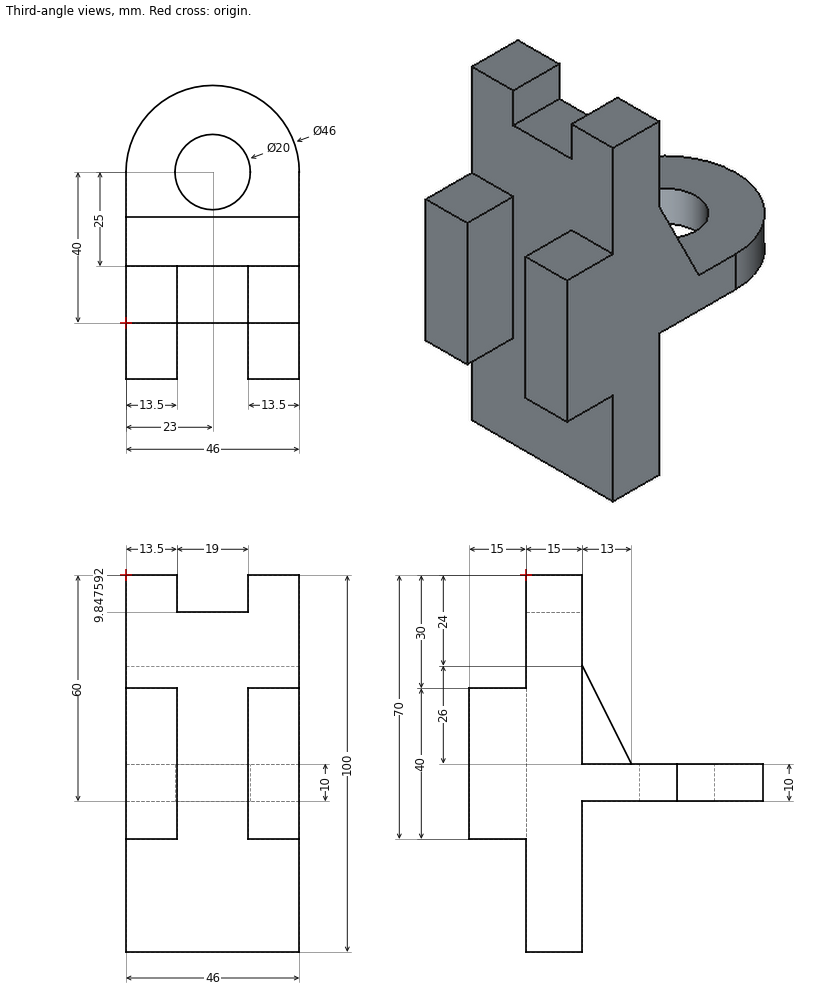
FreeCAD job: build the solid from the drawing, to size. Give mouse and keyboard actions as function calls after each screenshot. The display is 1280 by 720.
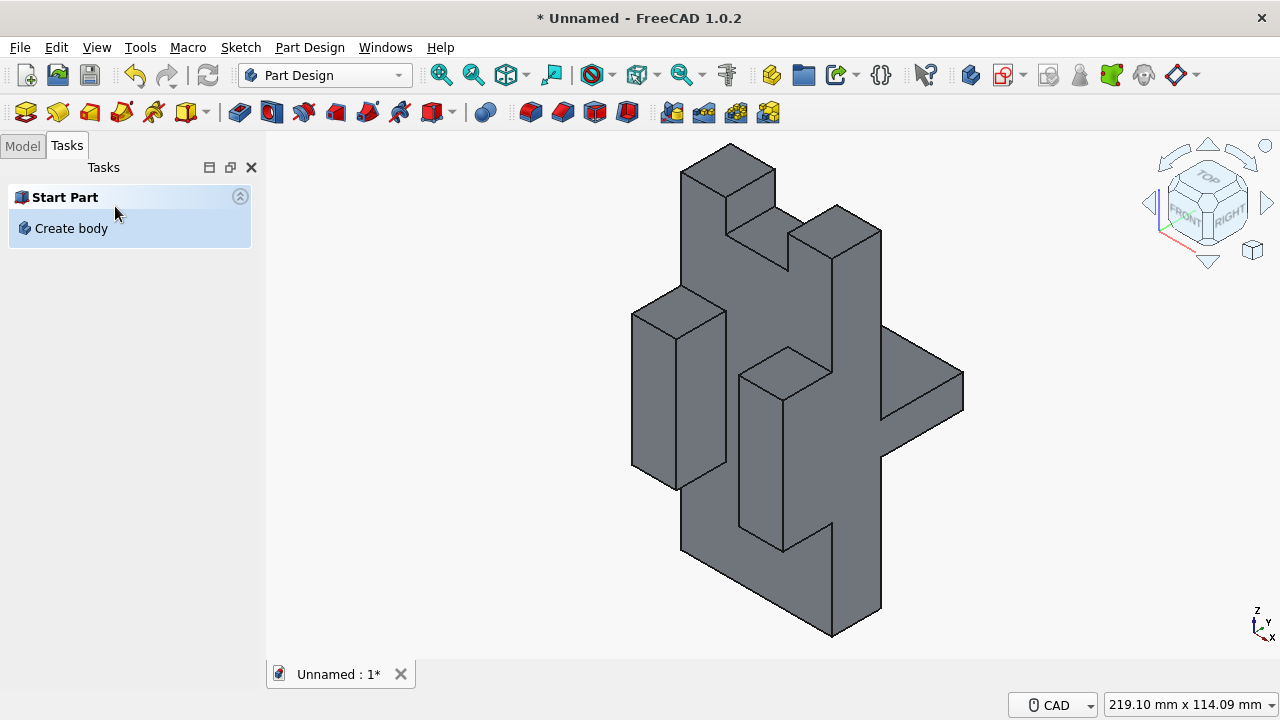
click(442, 76)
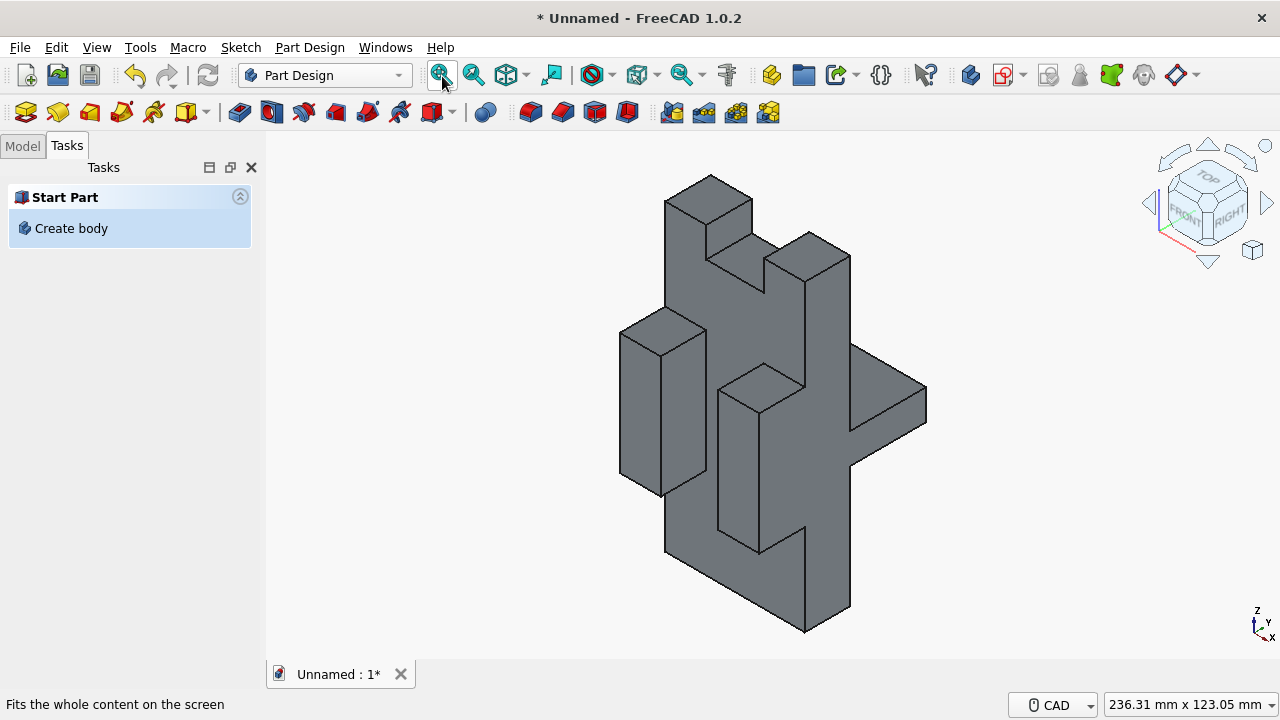
click(869, 384)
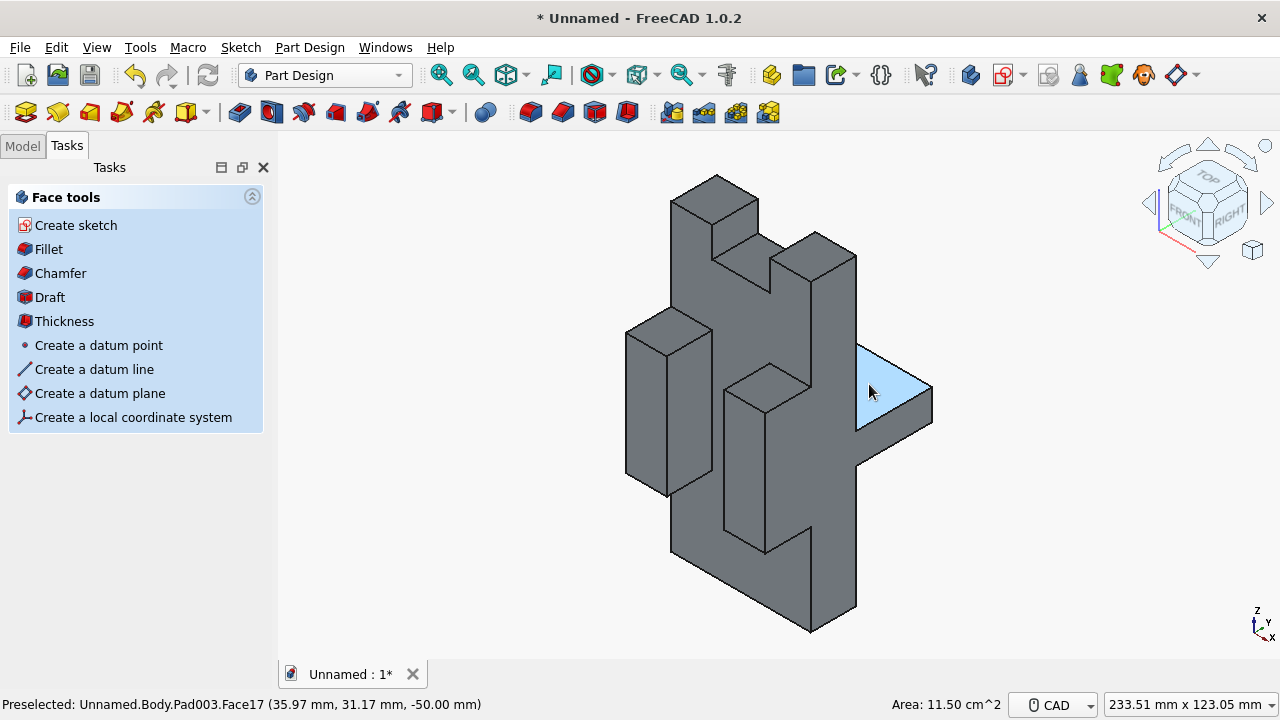
click(1004, 76)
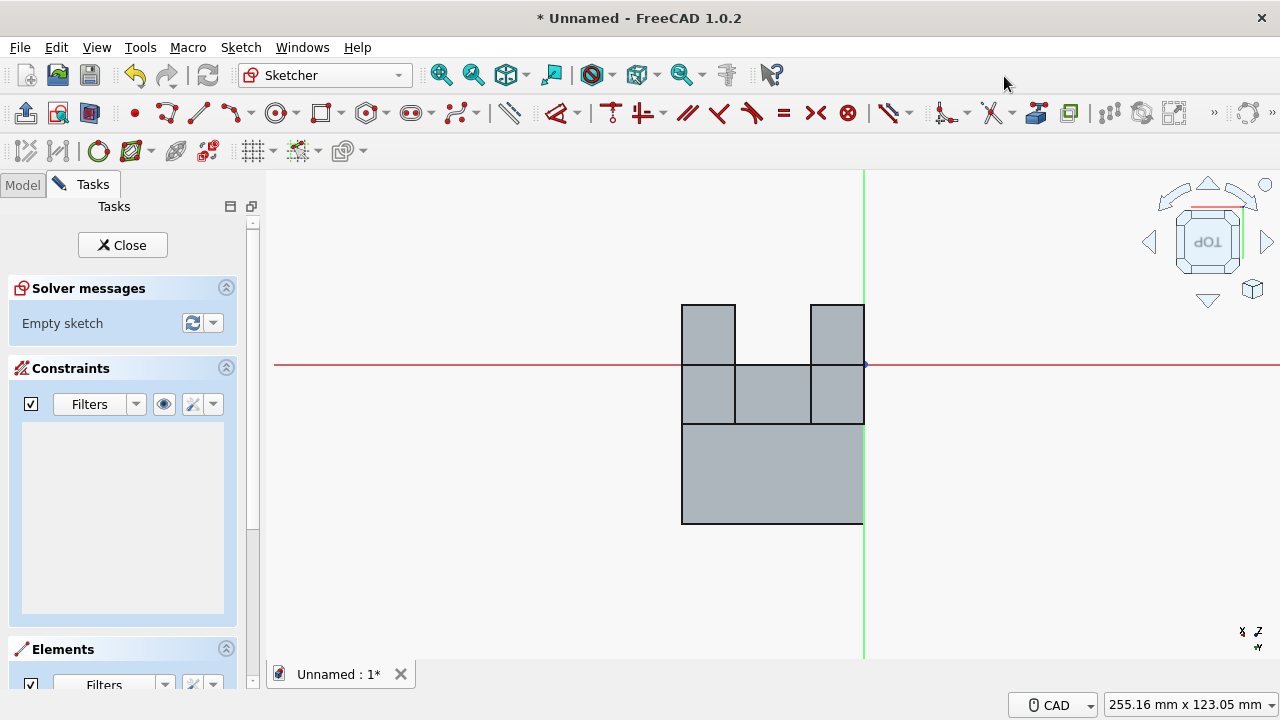
key(q)
key(s)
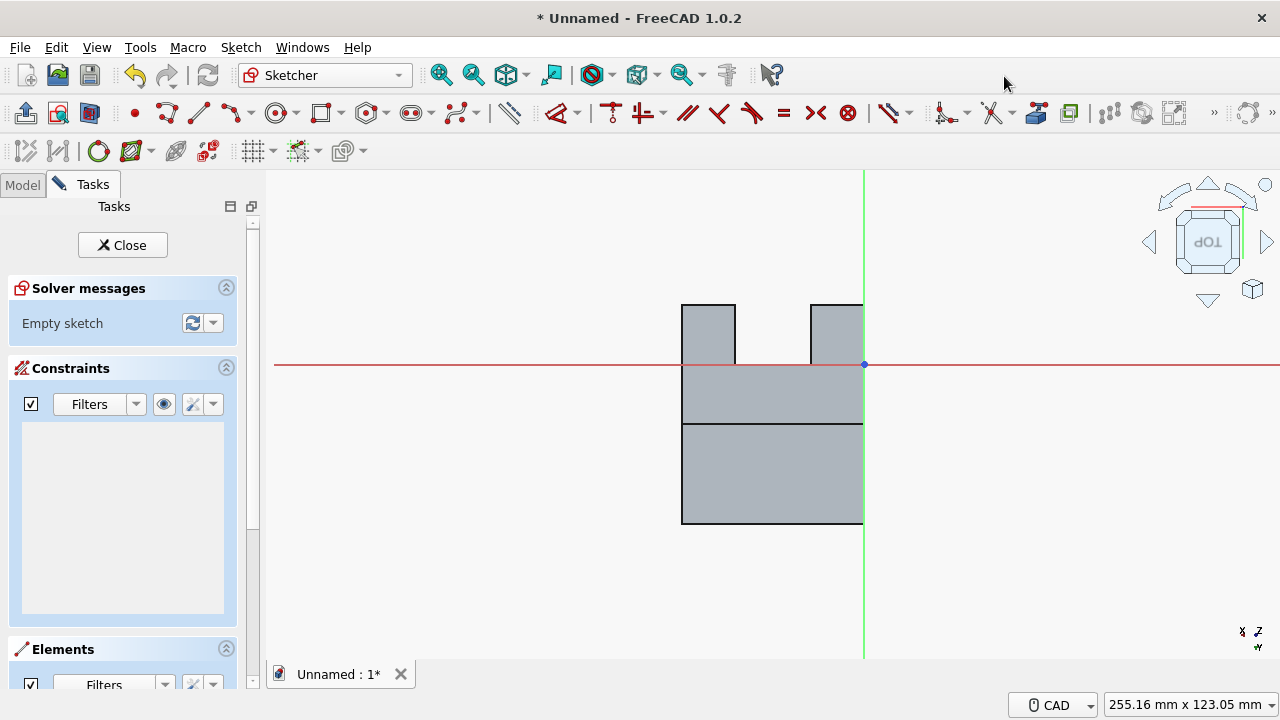
scroll(395, 198, down, 1)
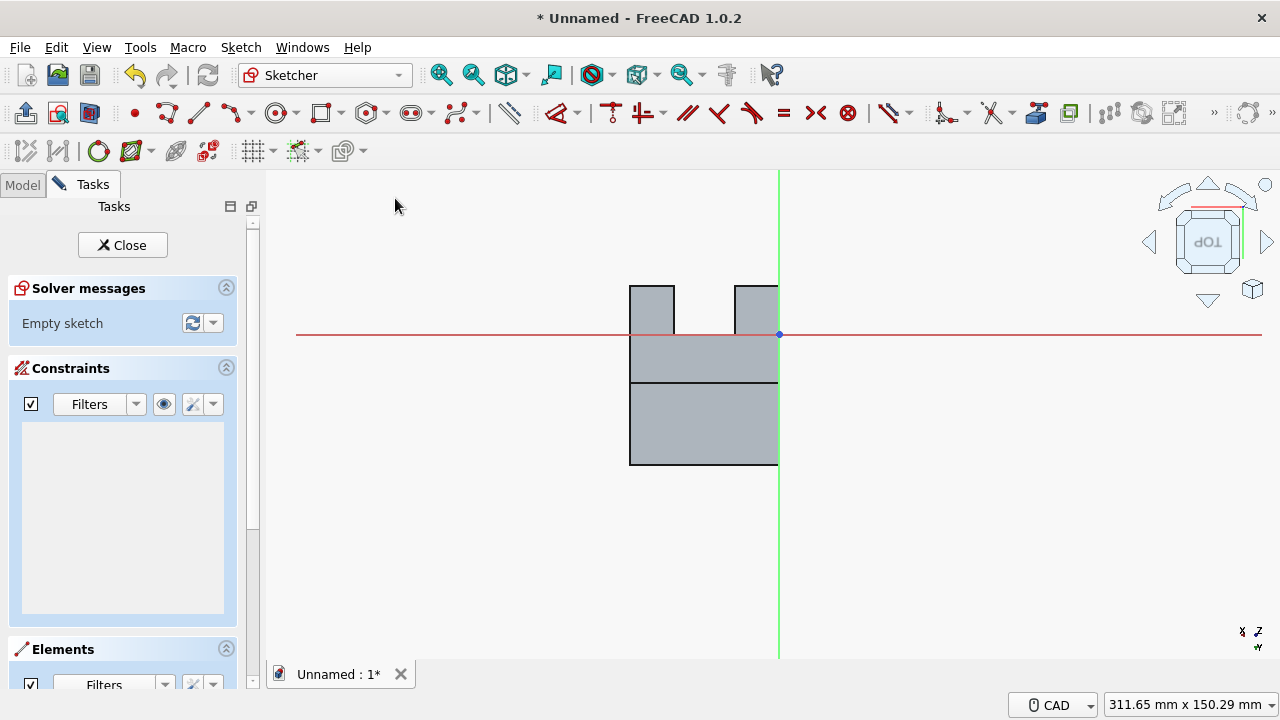
scroll(705, 483, up, 2)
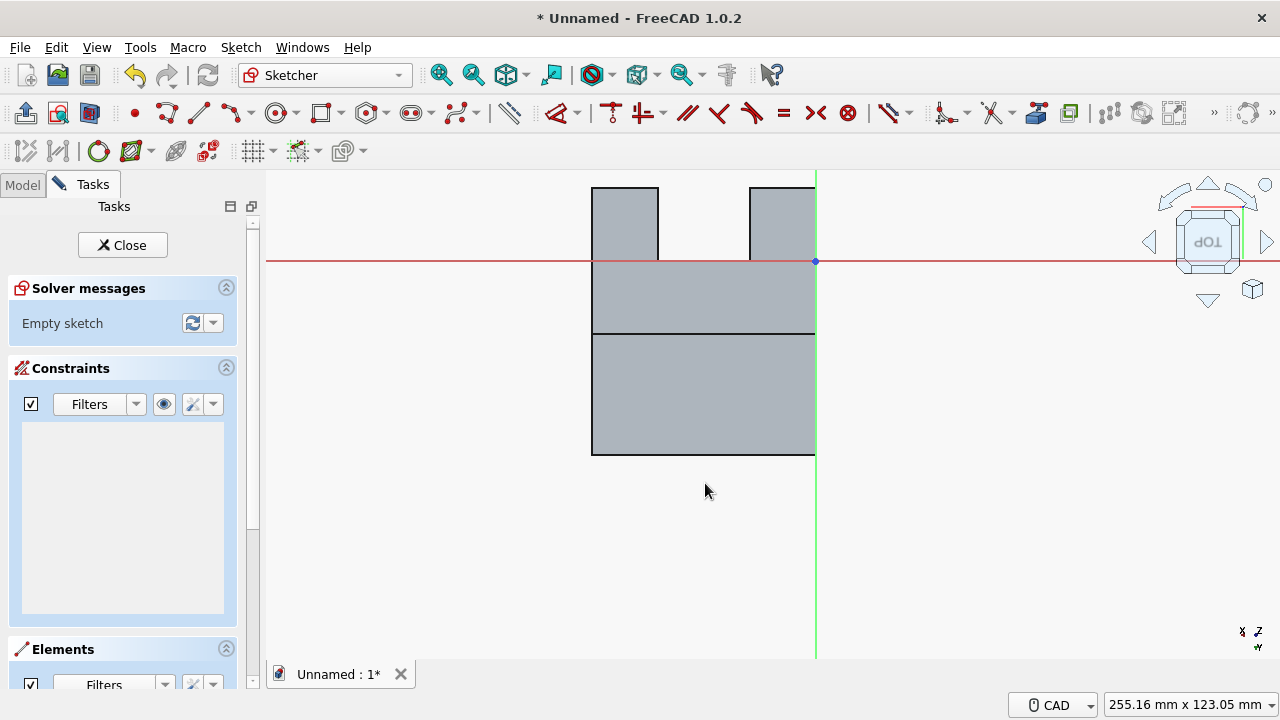
click(276, 114)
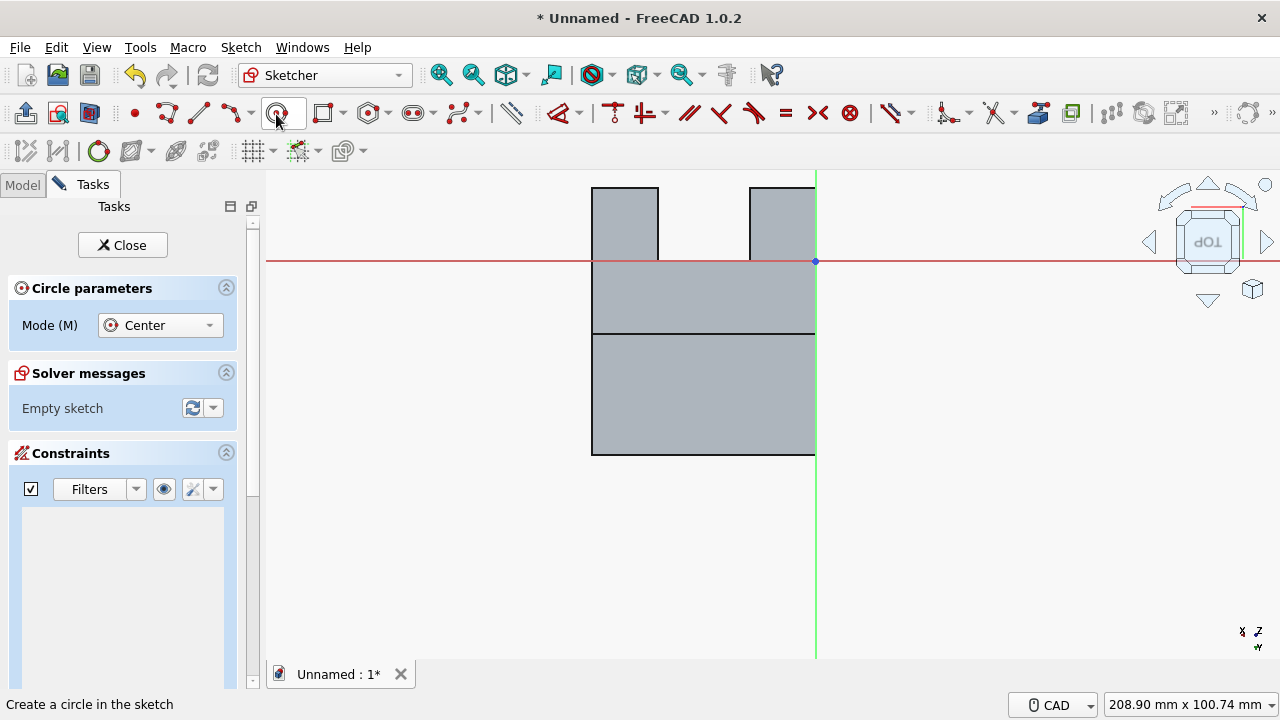
click(704, 455)
move(783, 377)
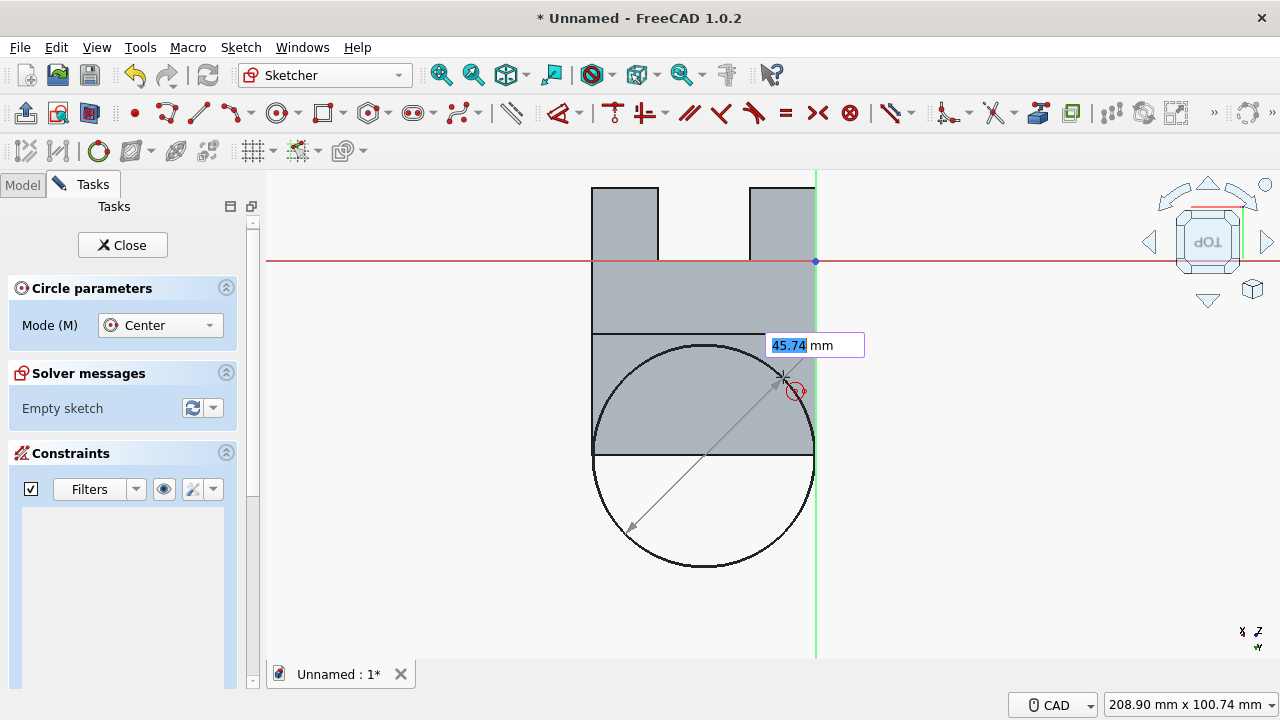
text(46)
key(Return)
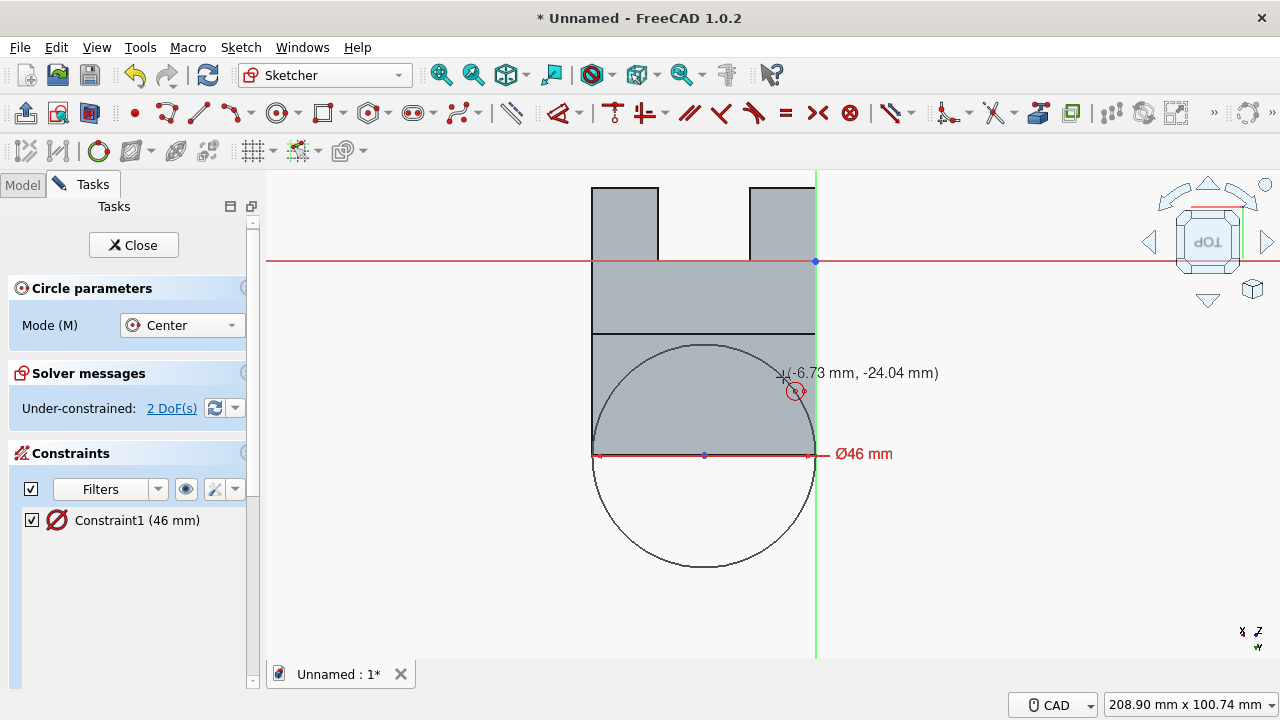
click(704, 456)
move(738, 421)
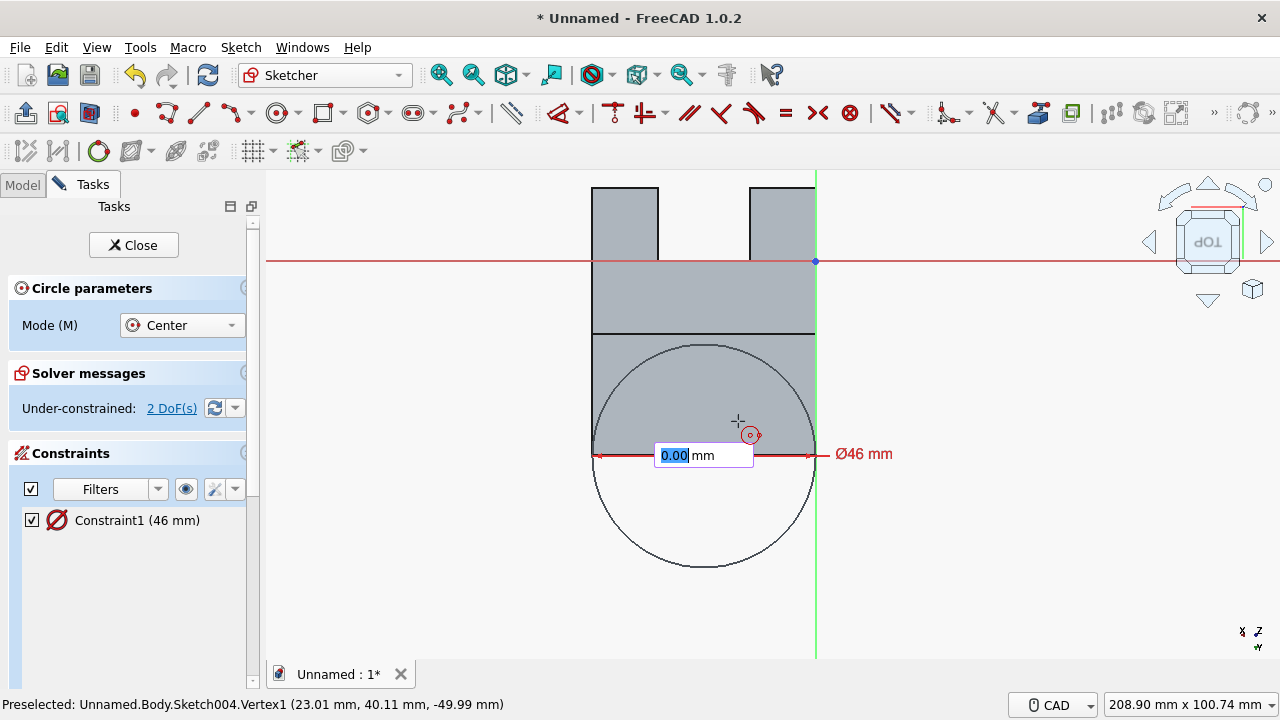
text(20)
key(Return)
key(Escape)